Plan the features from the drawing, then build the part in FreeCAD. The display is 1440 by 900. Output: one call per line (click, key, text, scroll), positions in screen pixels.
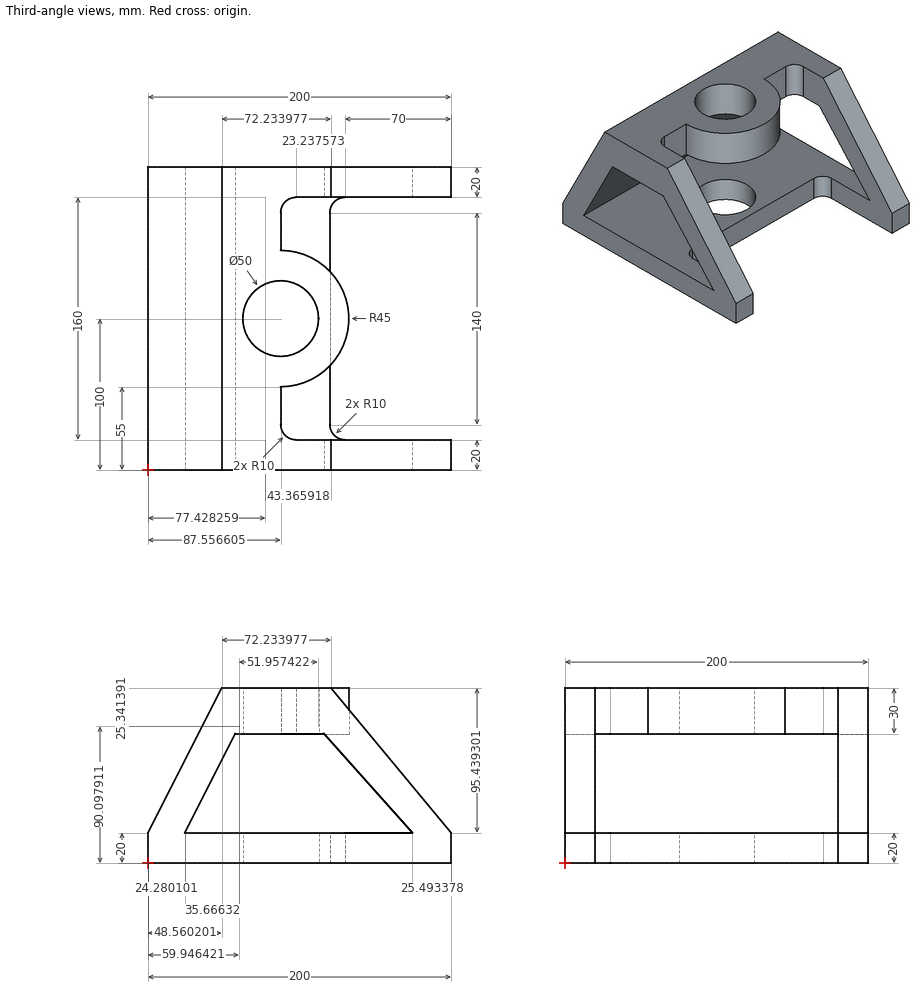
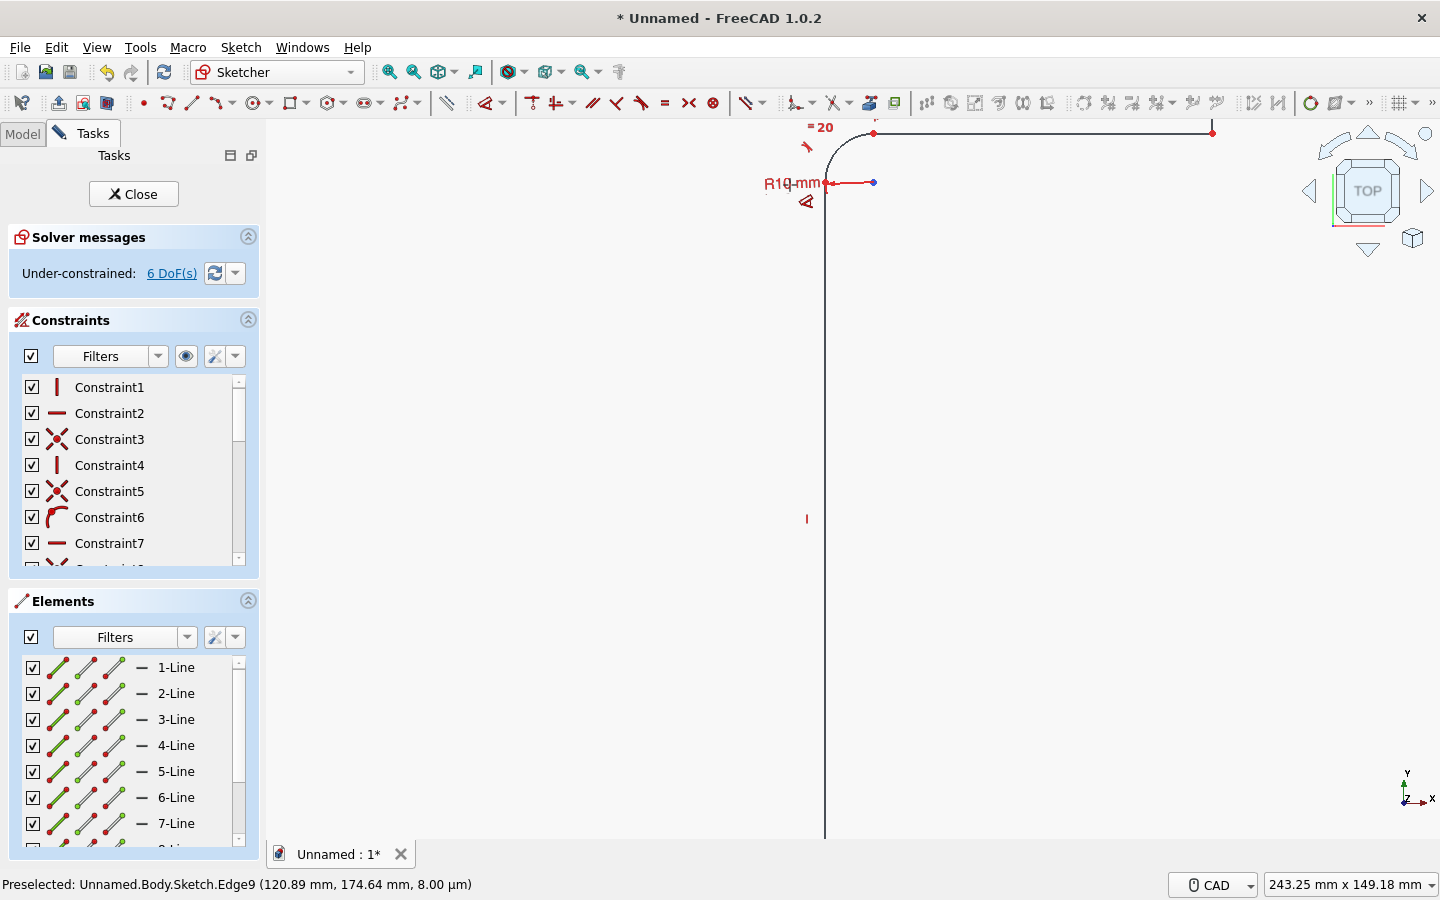
scroll(830, 448, down, 4)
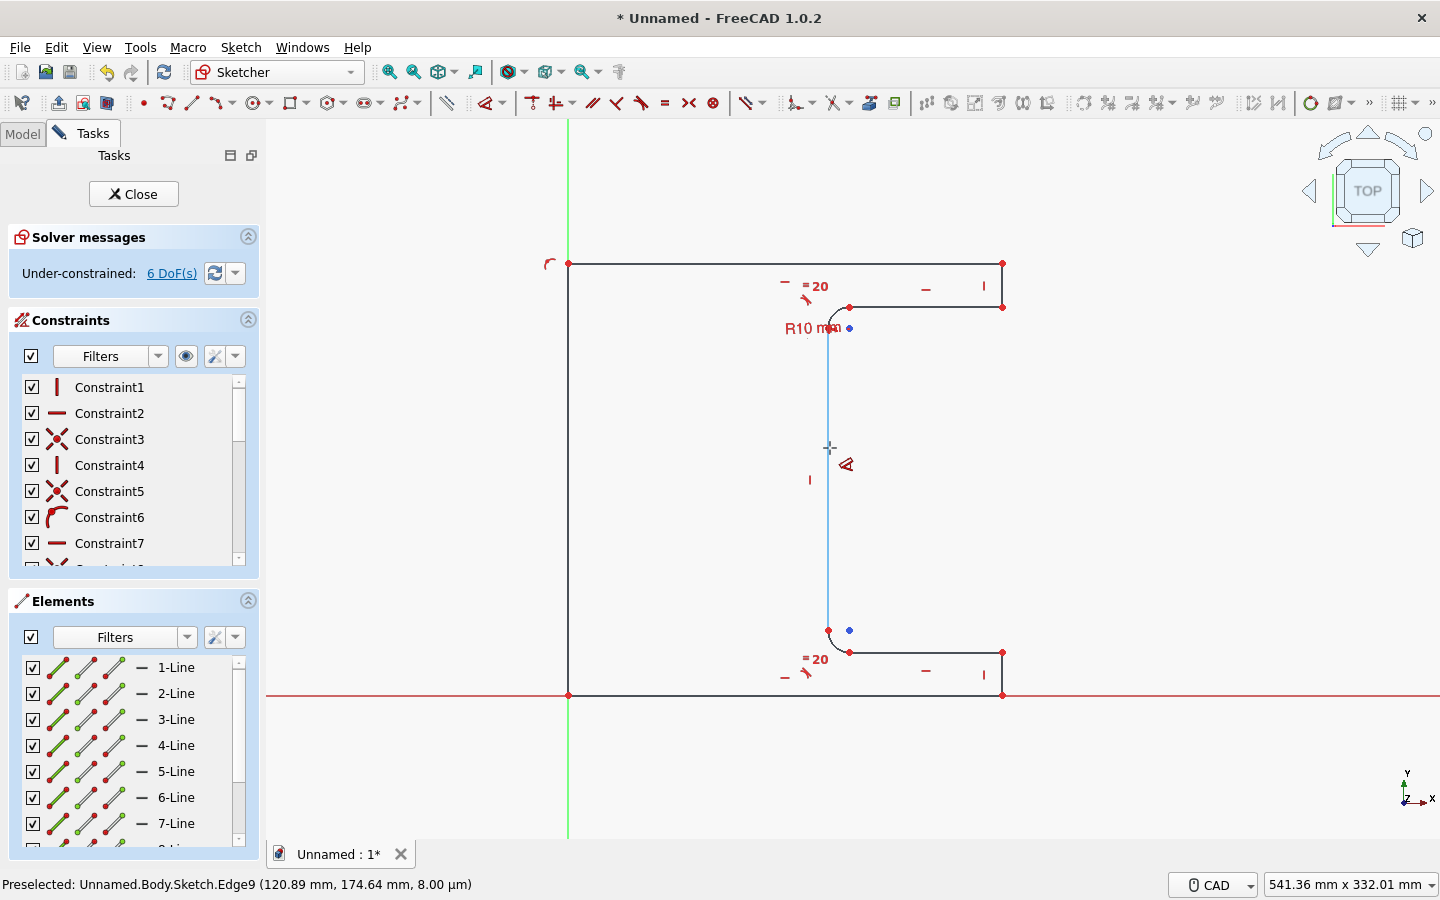
click(896, 307)
click(926, 341)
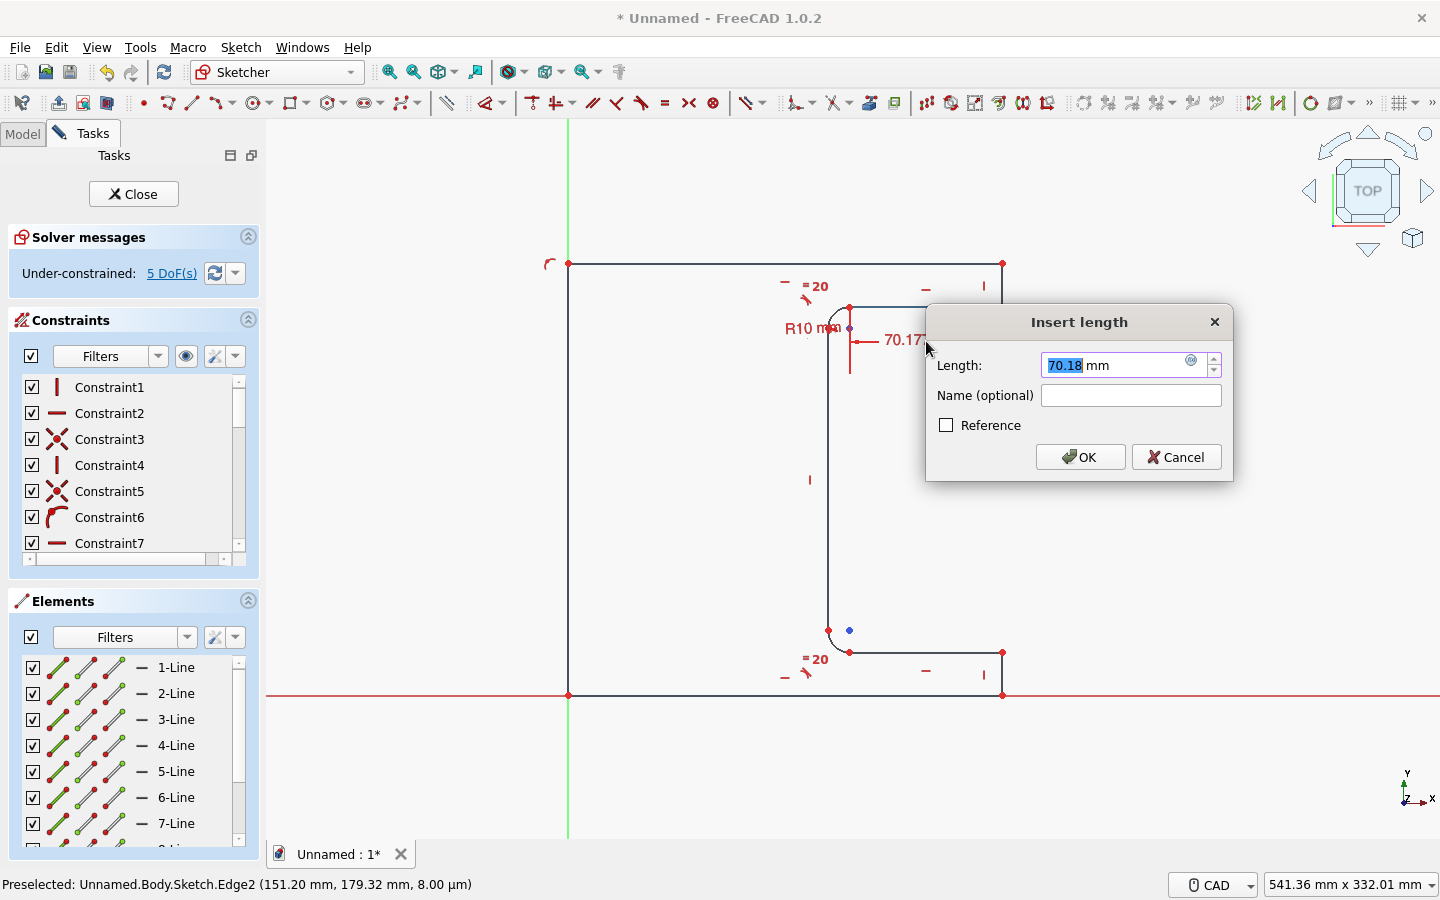
text(70)
key(Return)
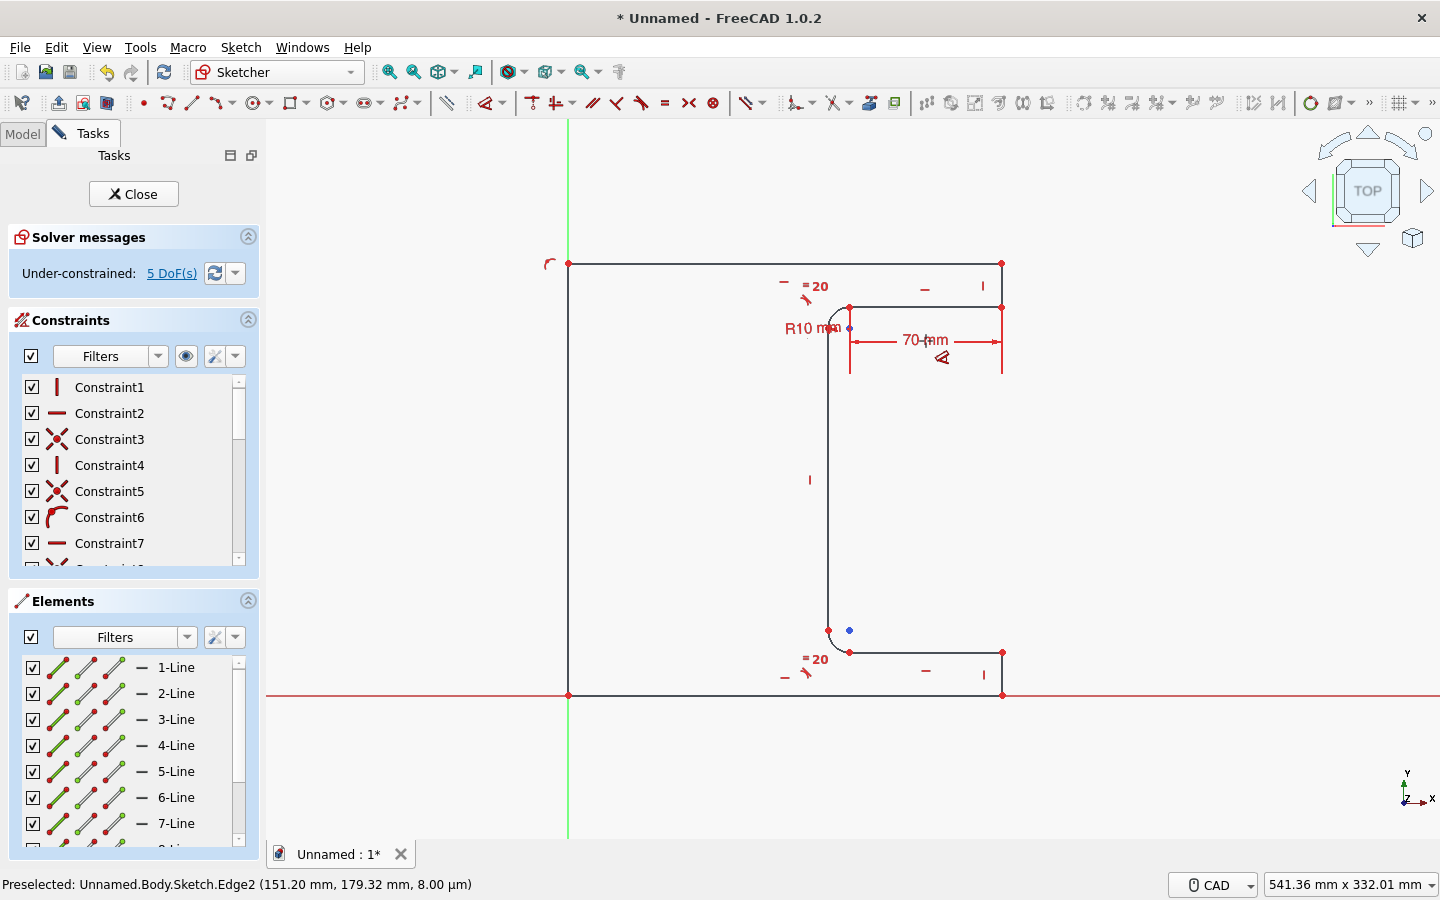
click(1002, 294)
click(1036, 285)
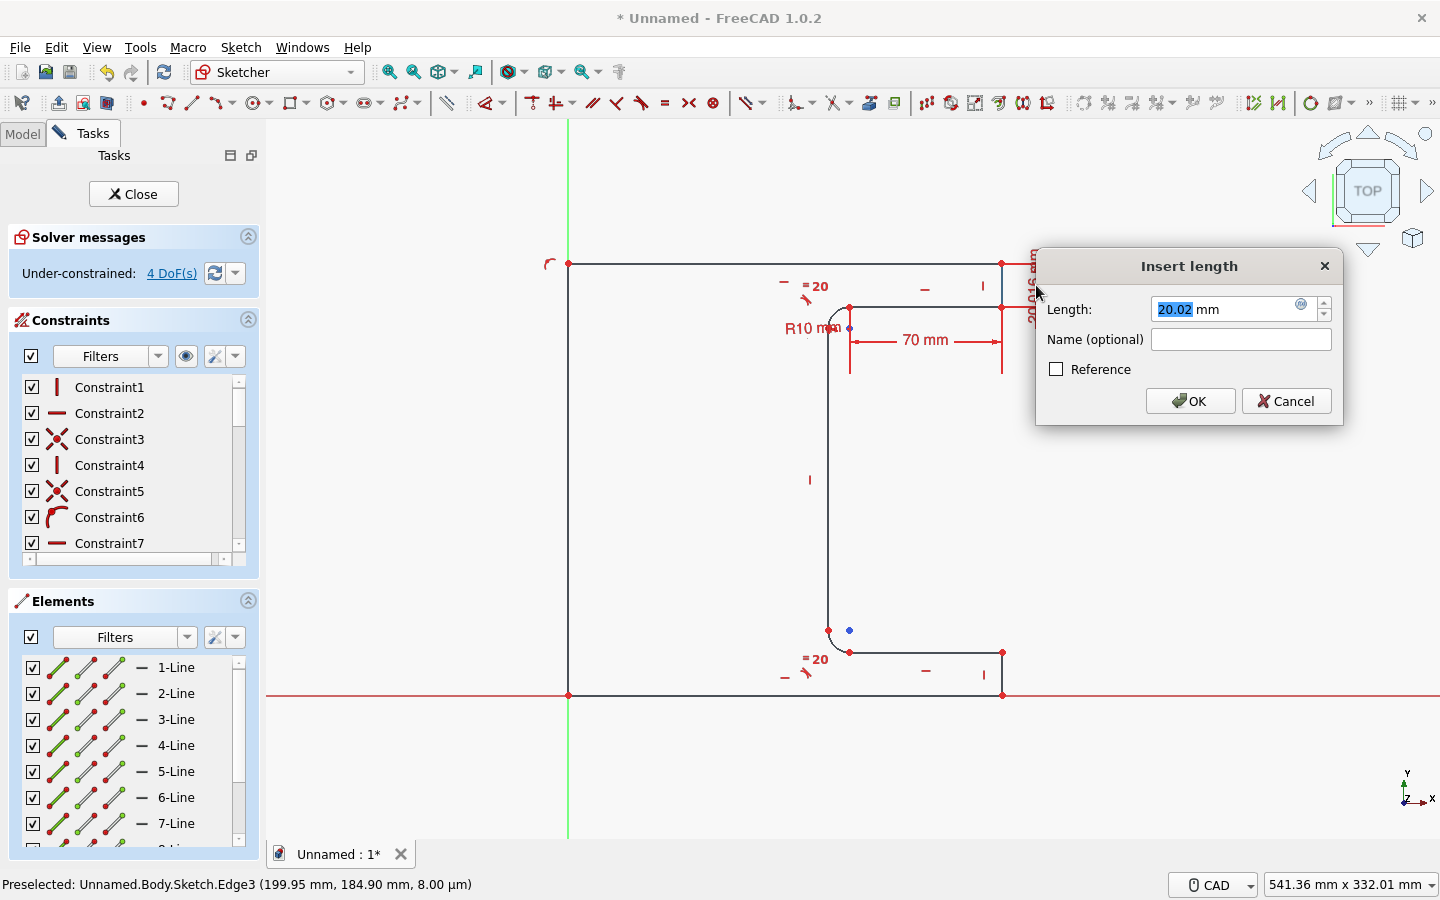
text(20)
key(Return)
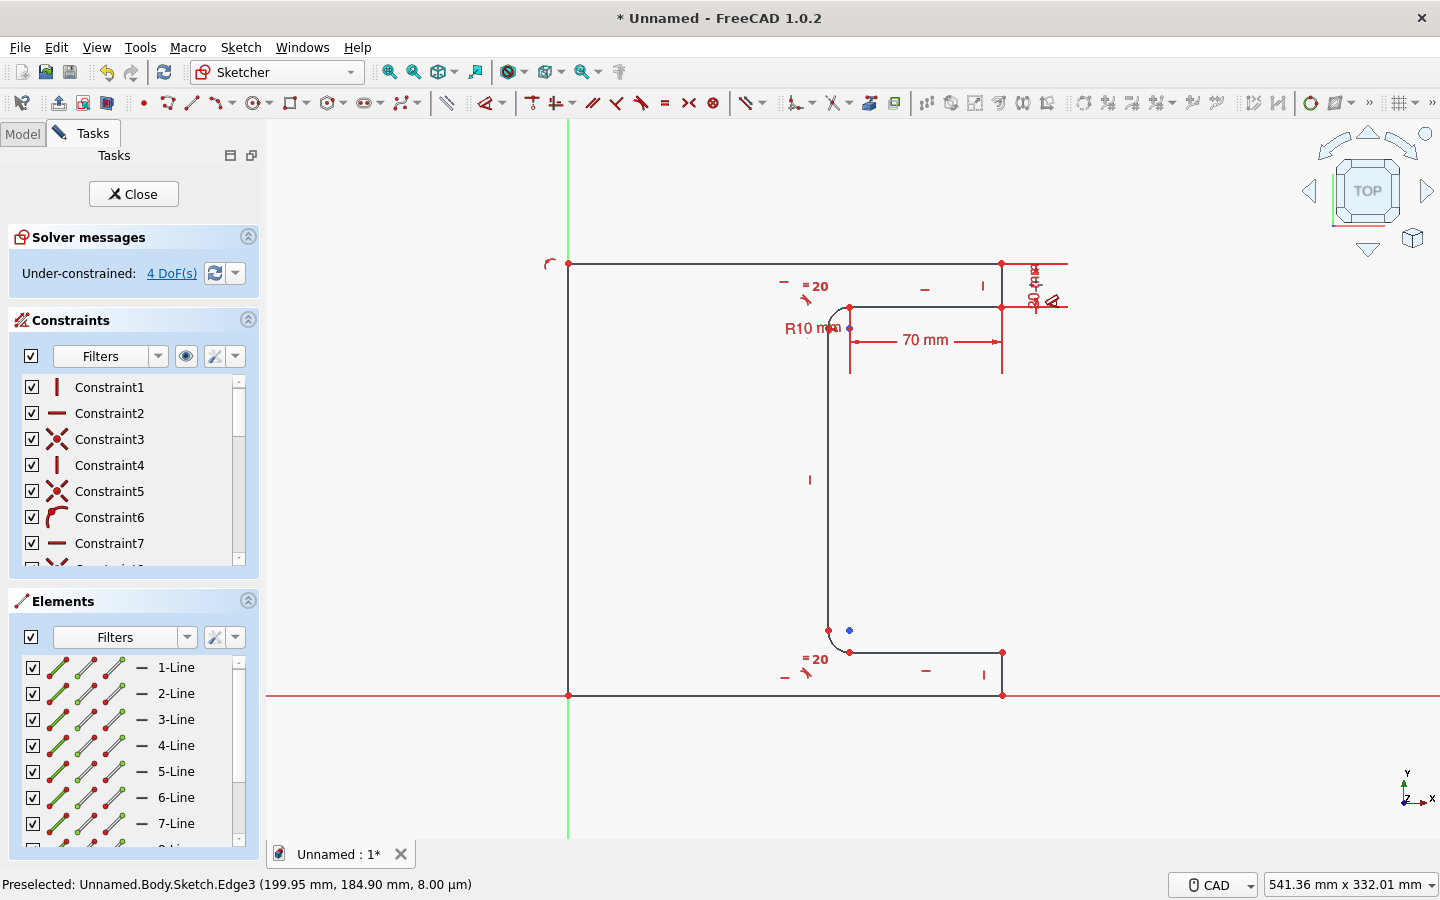
click(1002, 683)
click(1036, 674)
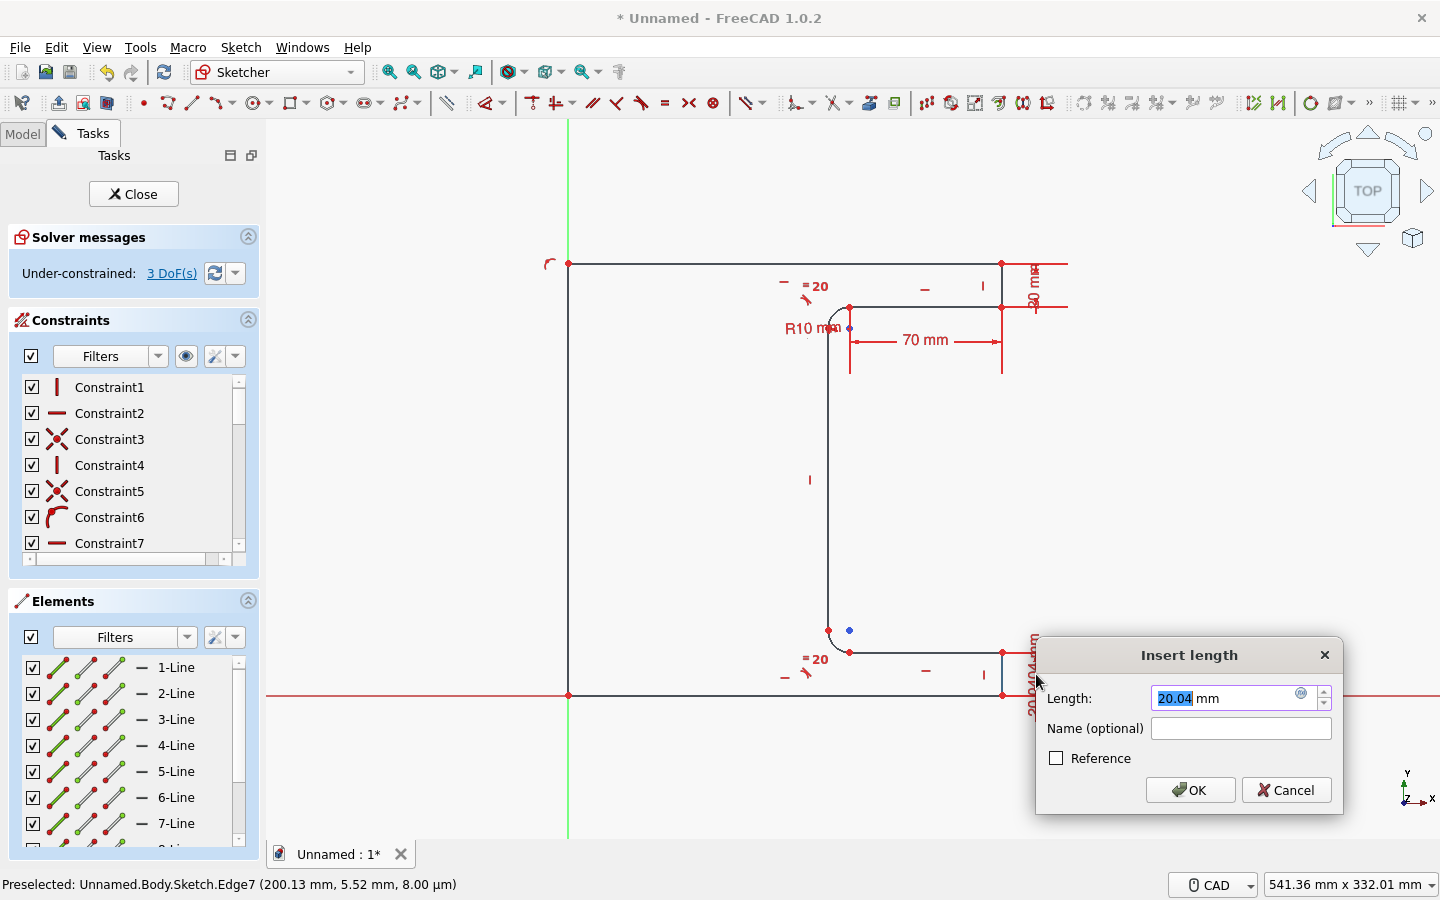
text(20)
key(Return)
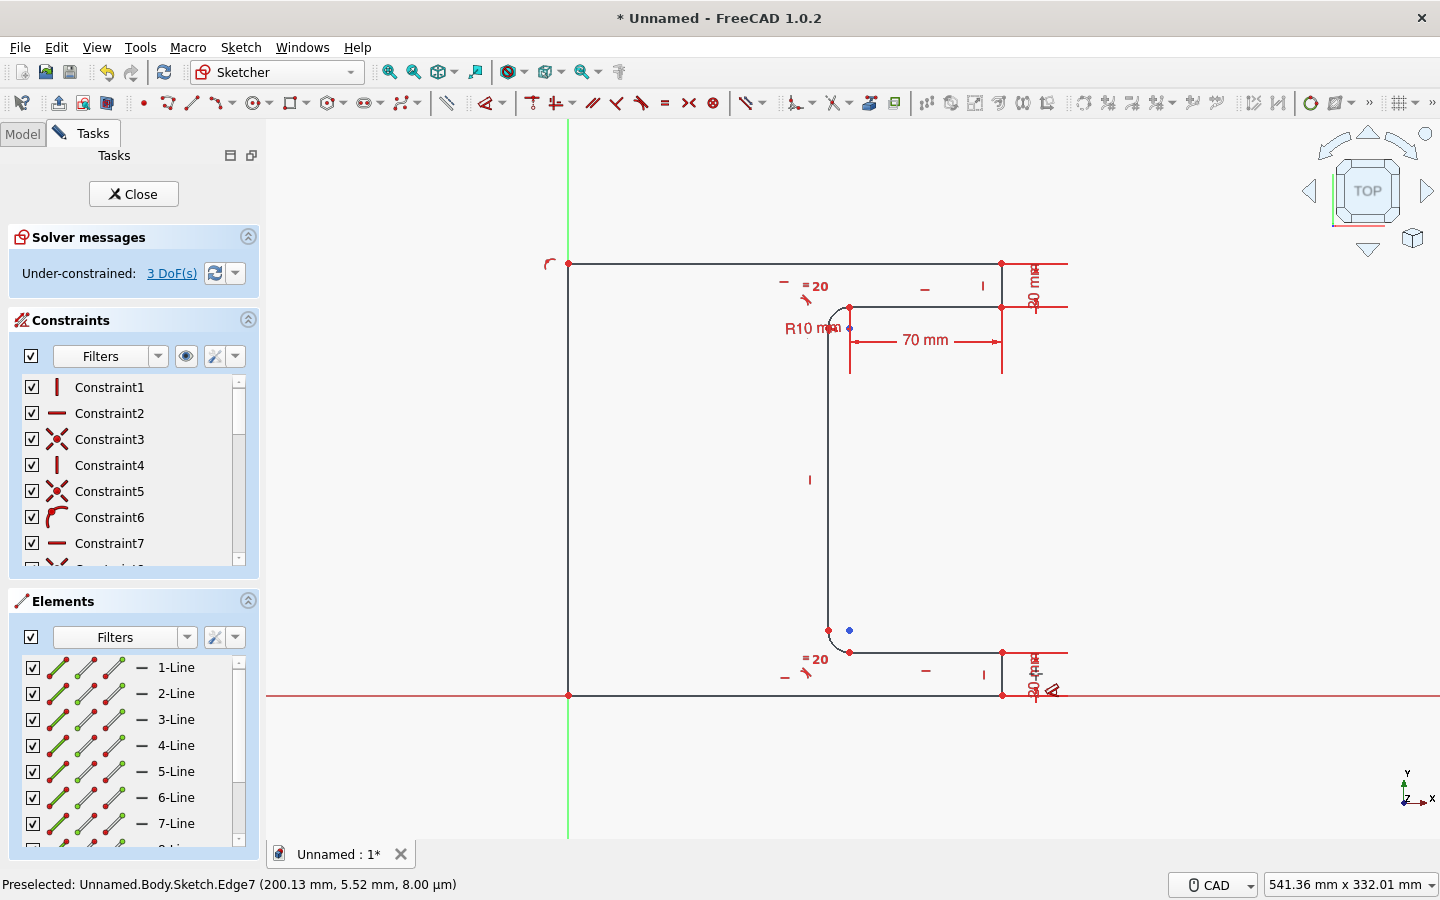
click(956, 653)
click(926, 619)